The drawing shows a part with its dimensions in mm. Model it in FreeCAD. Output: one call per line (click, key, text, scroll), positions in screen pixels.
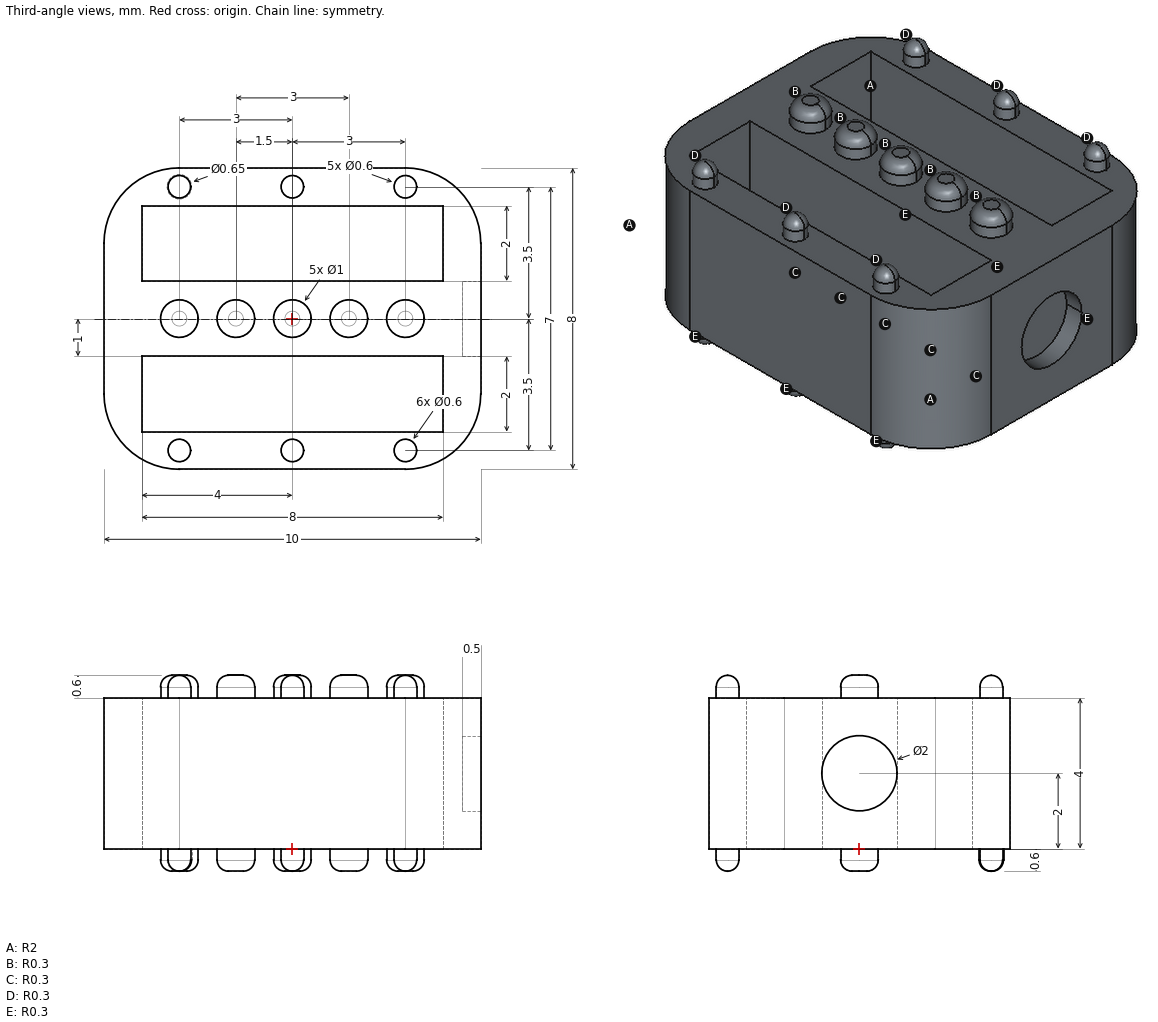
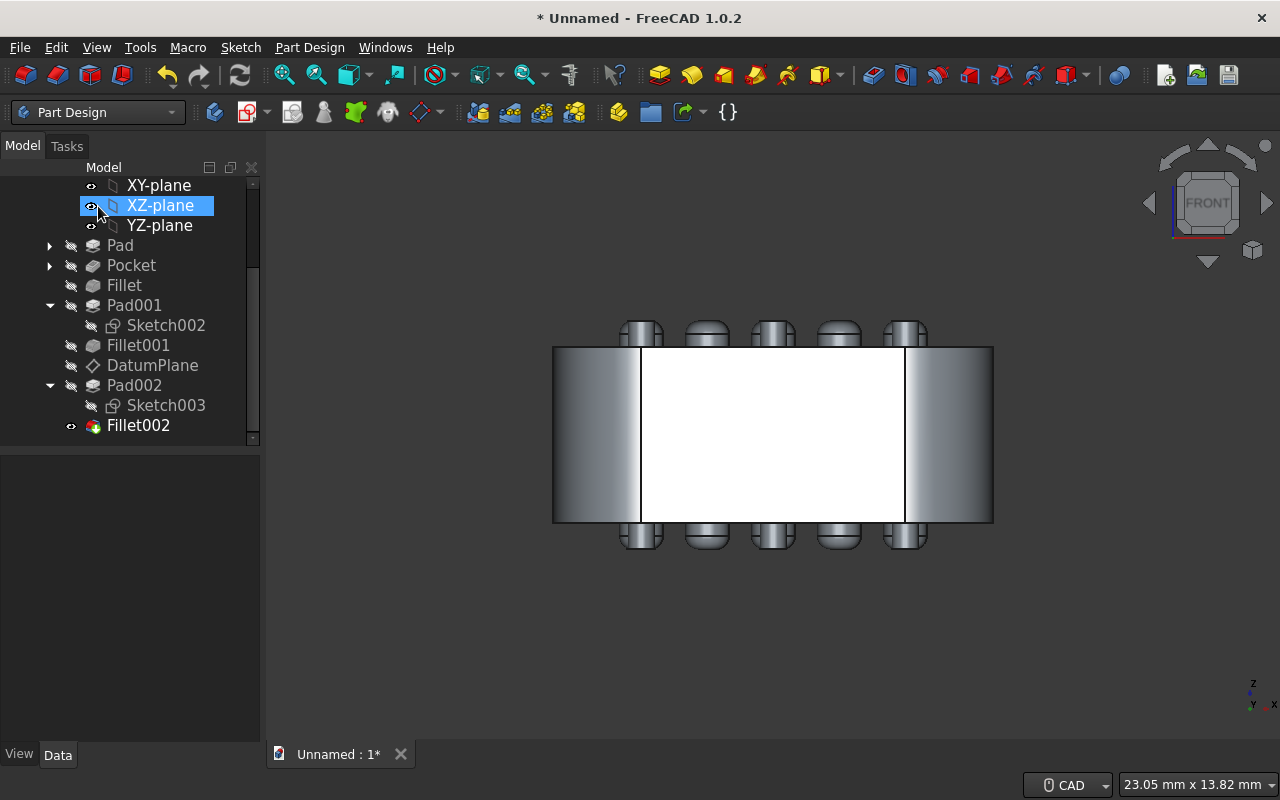
click(286, 76)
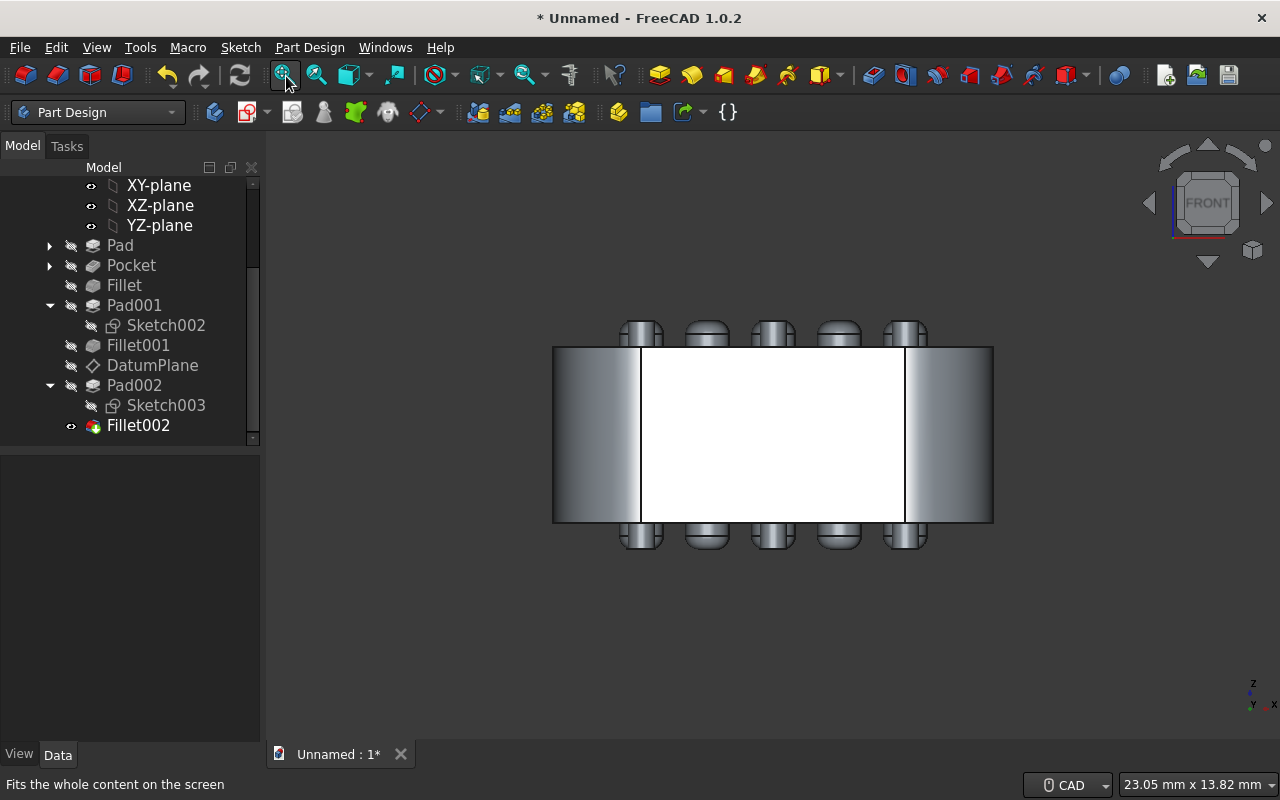
click(892, 320)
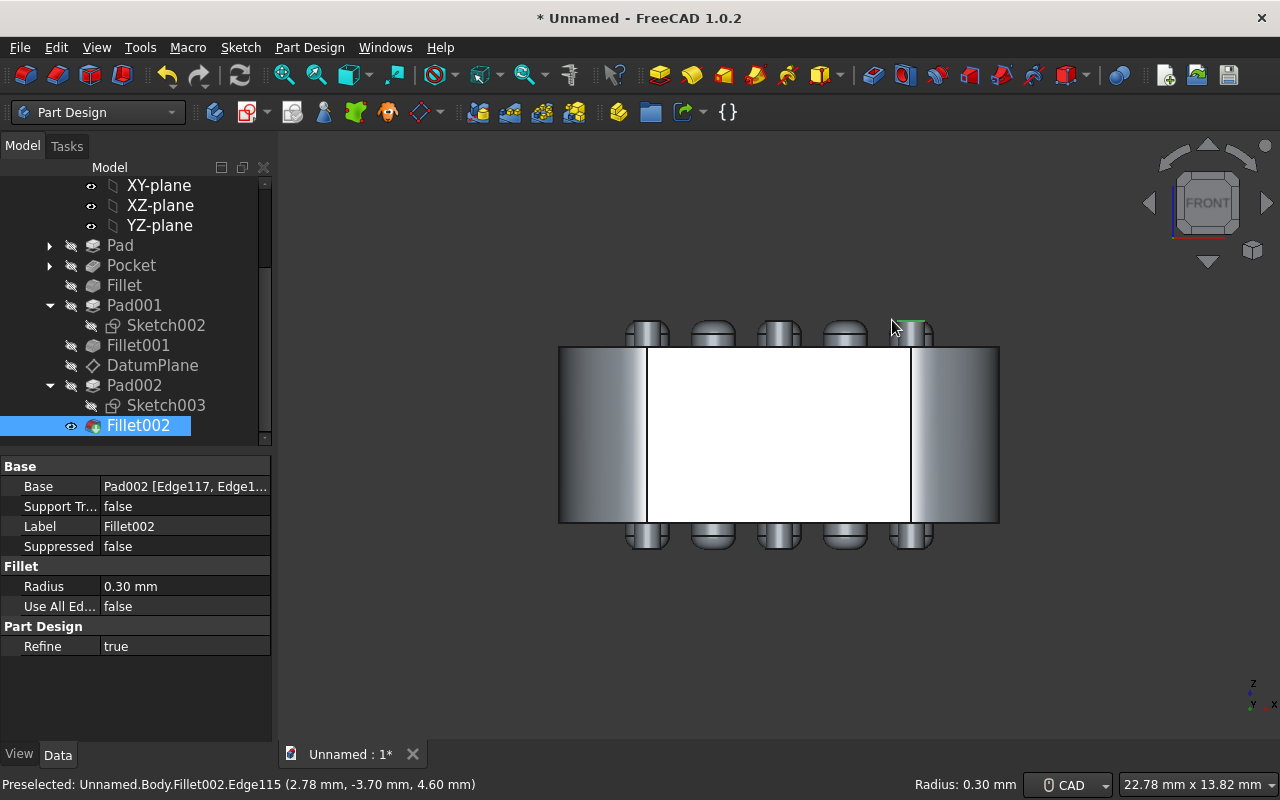
click(766, 320, ctrl)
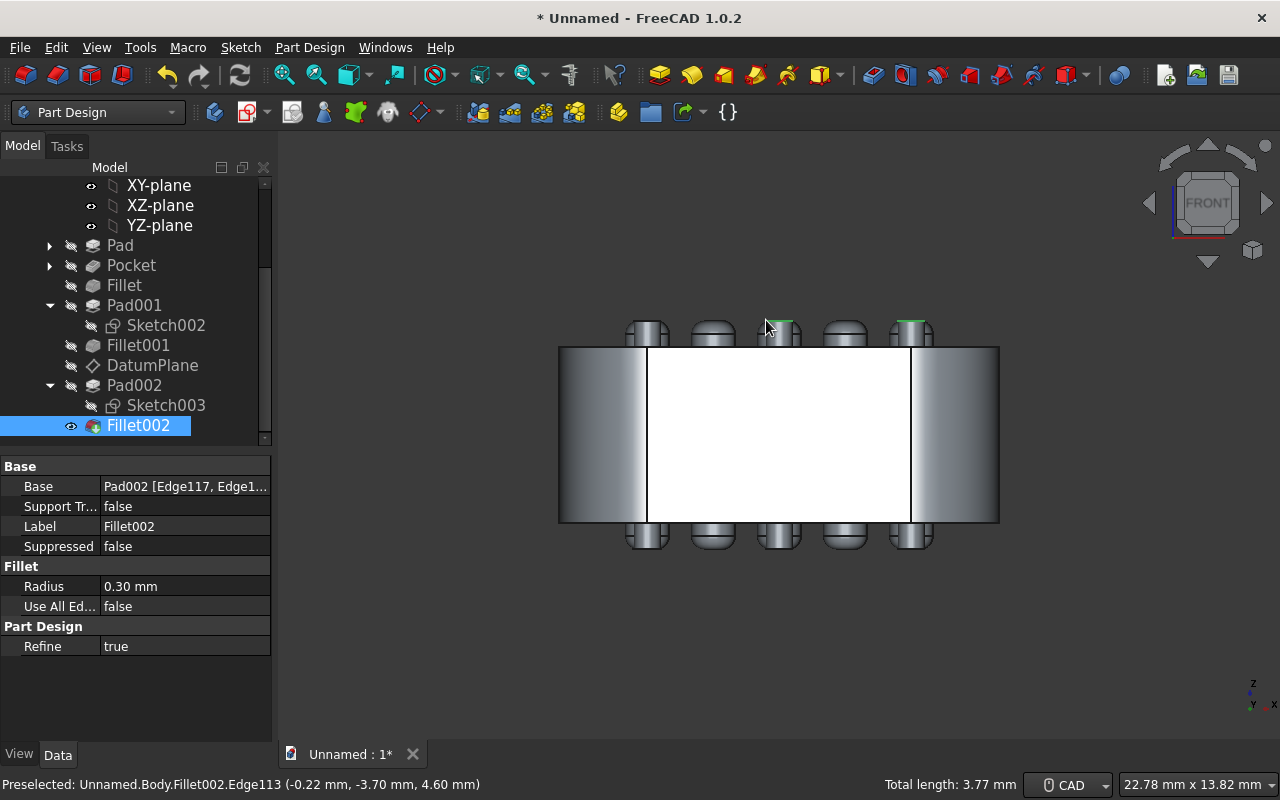
click(634, 320, ctrl)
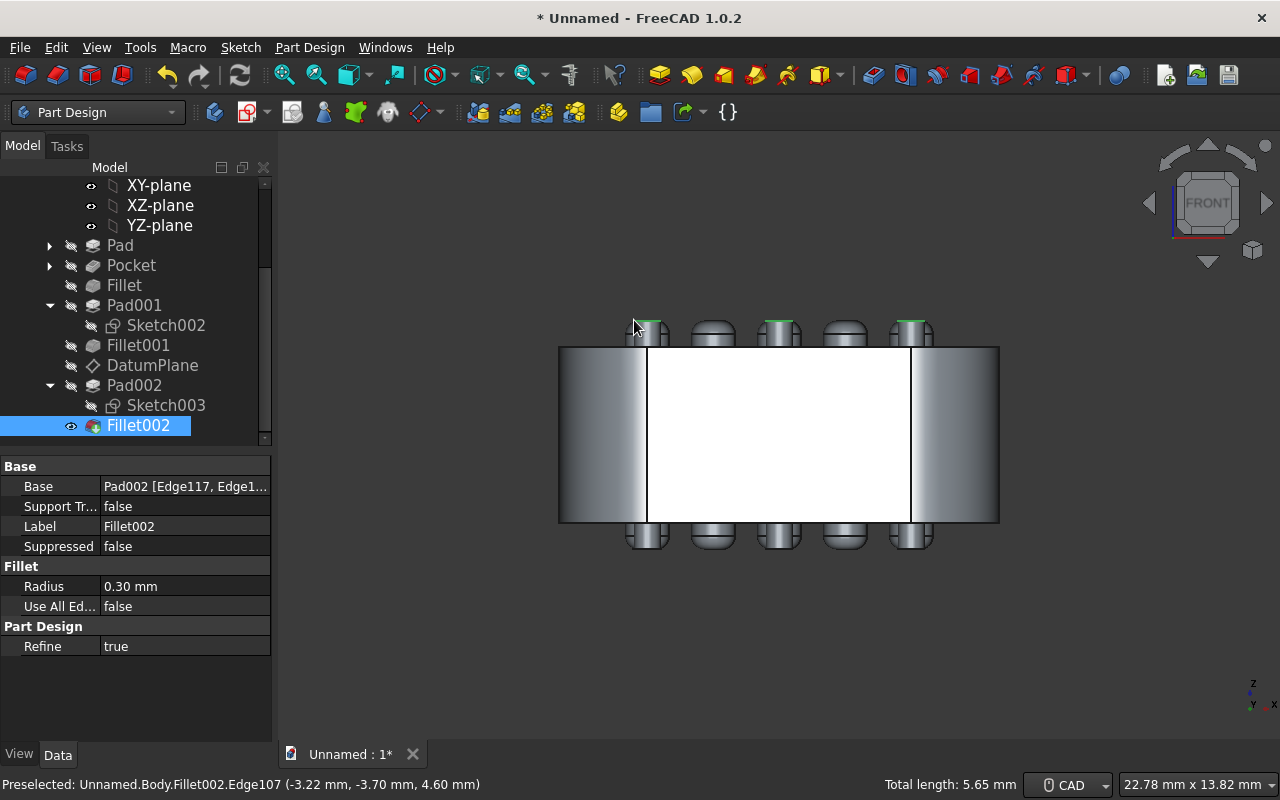
key(0)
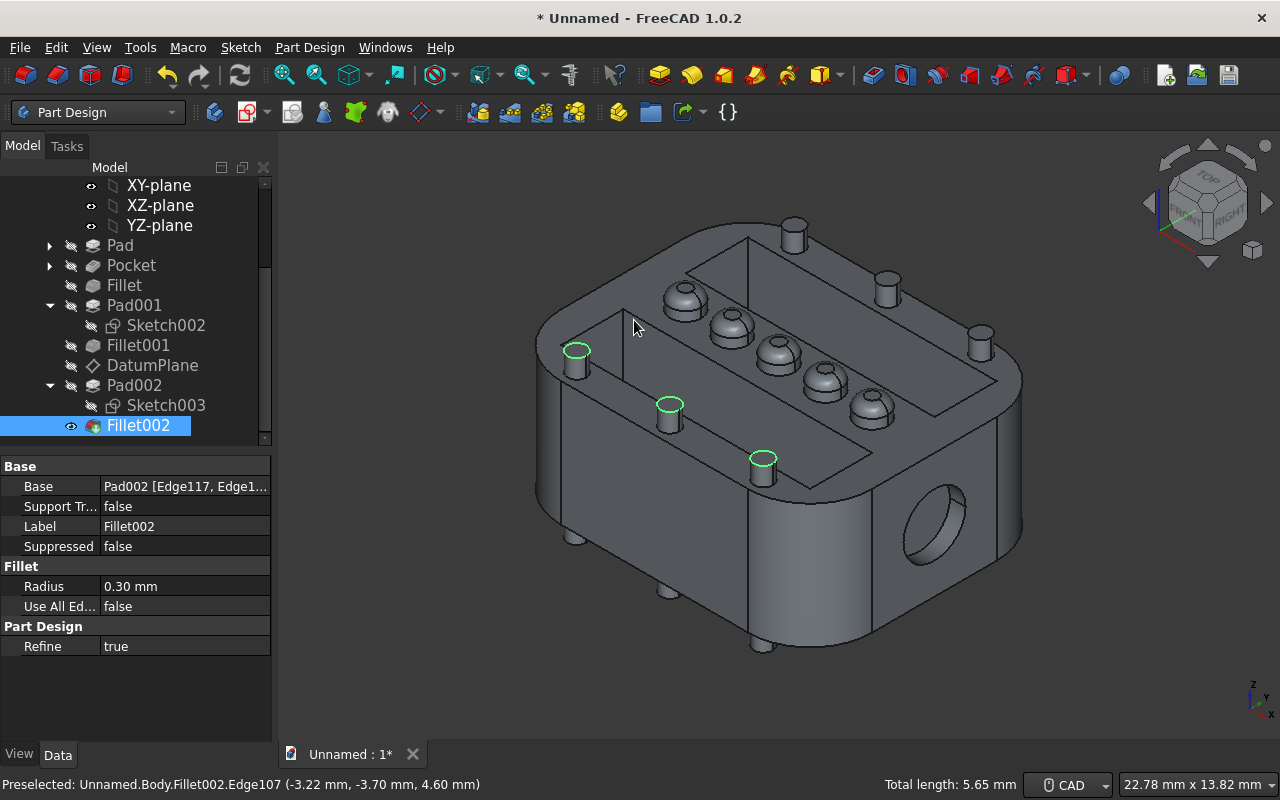
click(879, 272, ctrl)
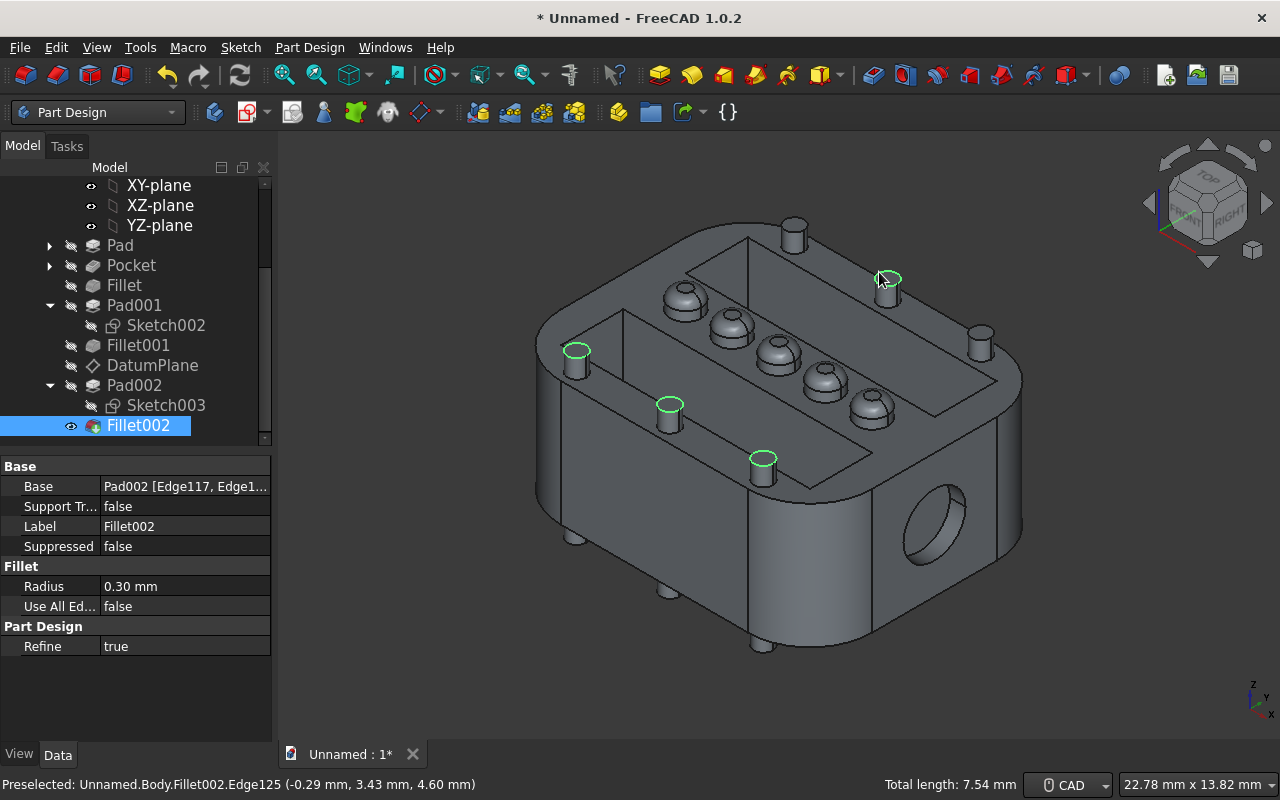
click(782, 223, ctrl)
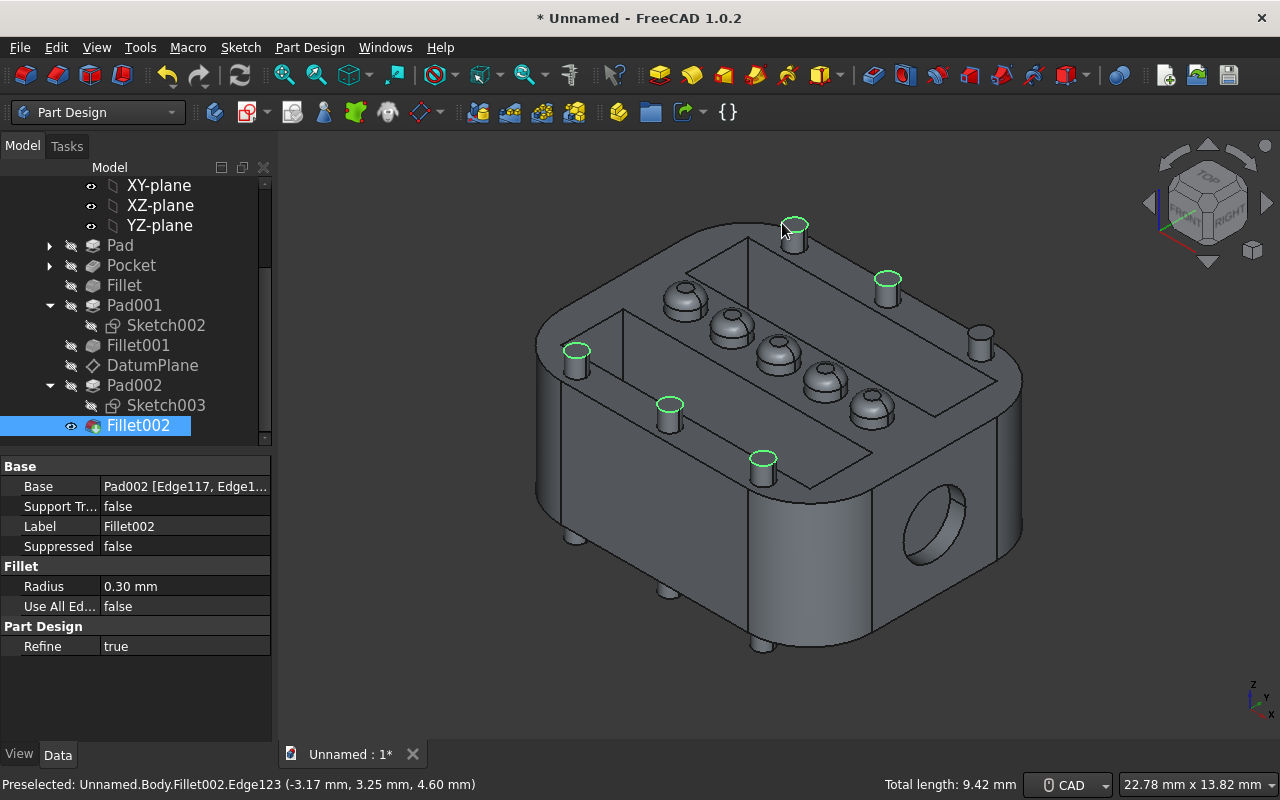
click(972, 326, ctrl)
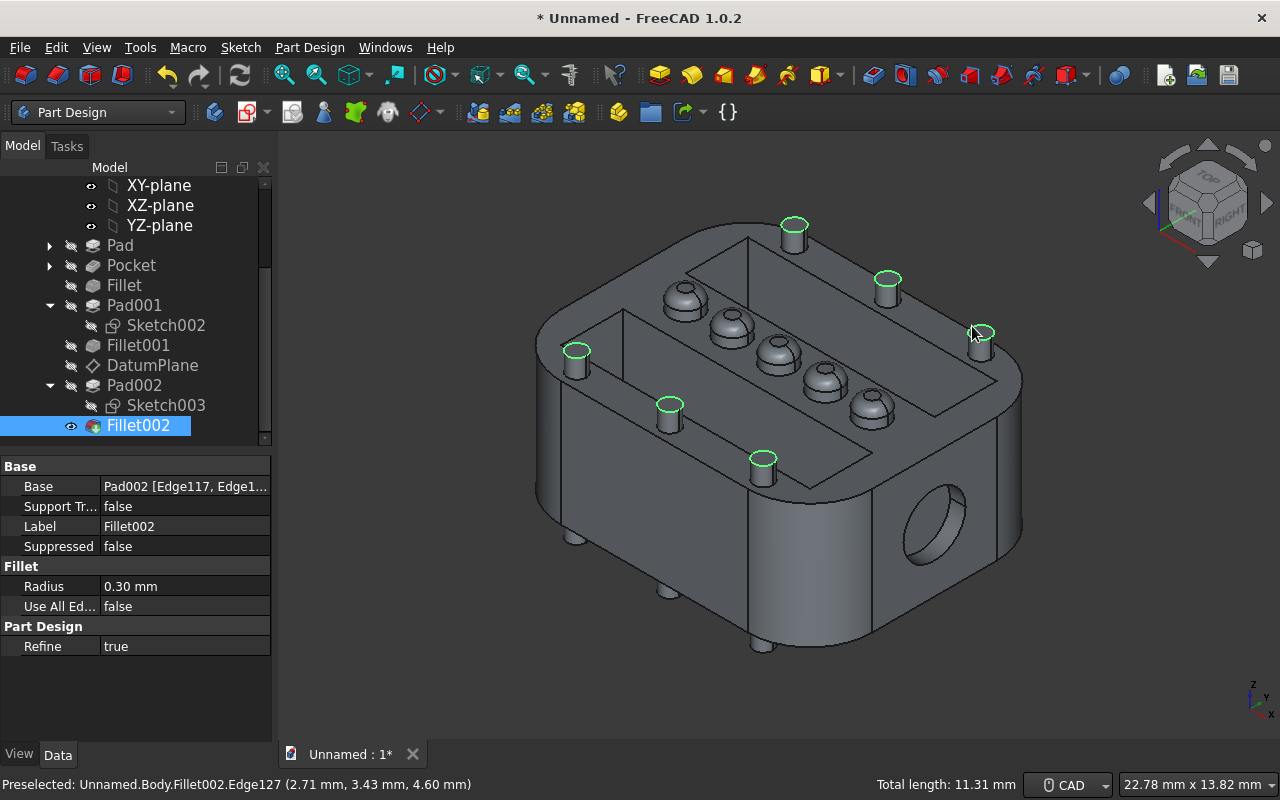
click(26, 76)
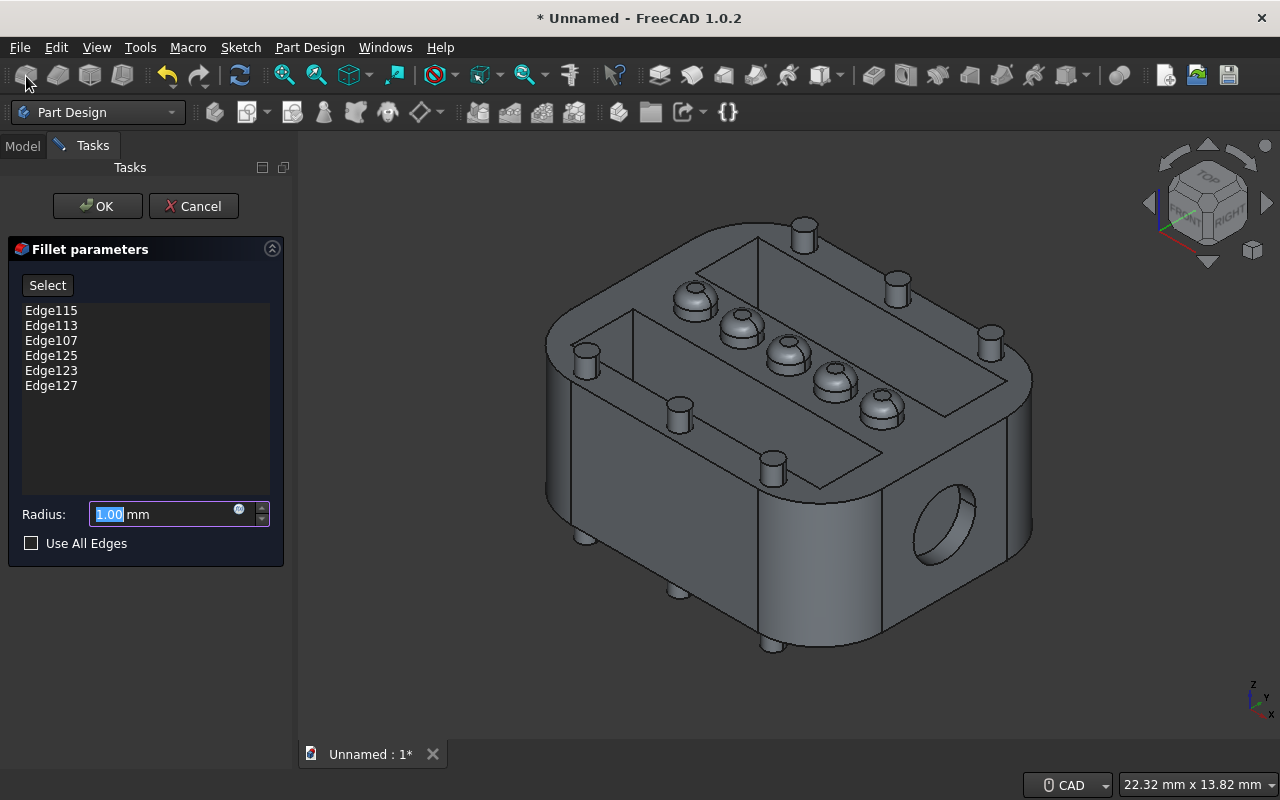
text(0.3)
key(Tab)